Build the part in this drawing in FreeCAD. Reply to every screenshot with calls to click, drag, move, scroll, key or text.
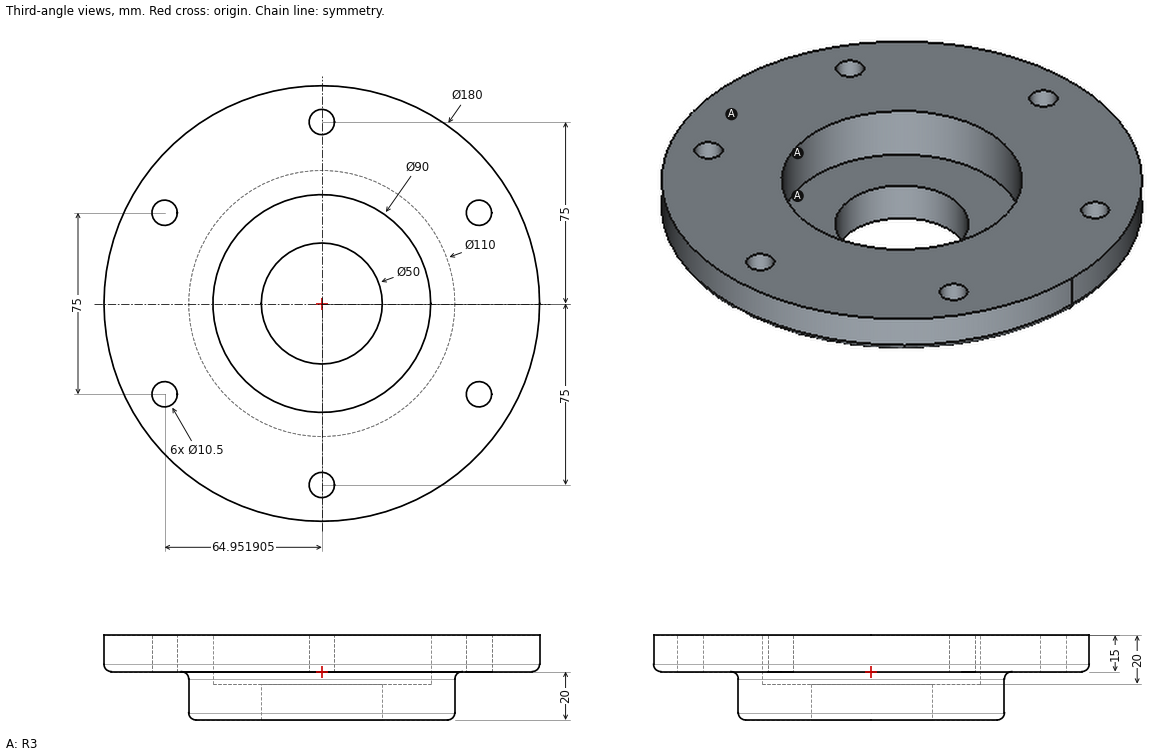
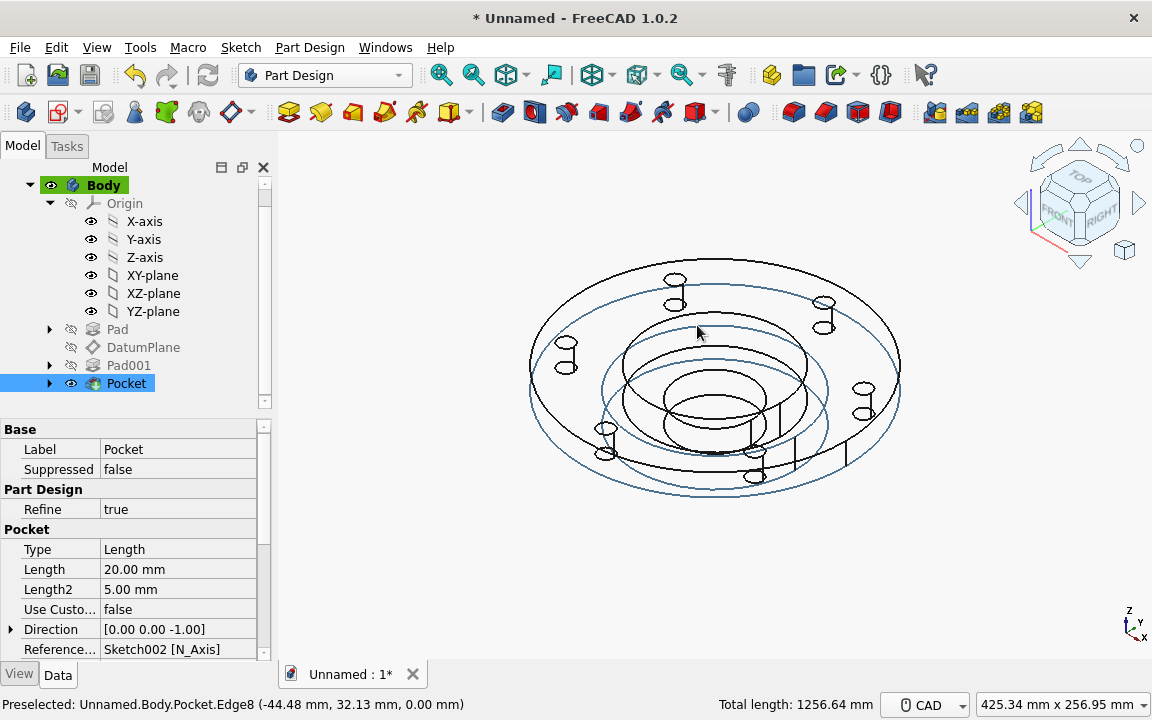
key(v)
key(1)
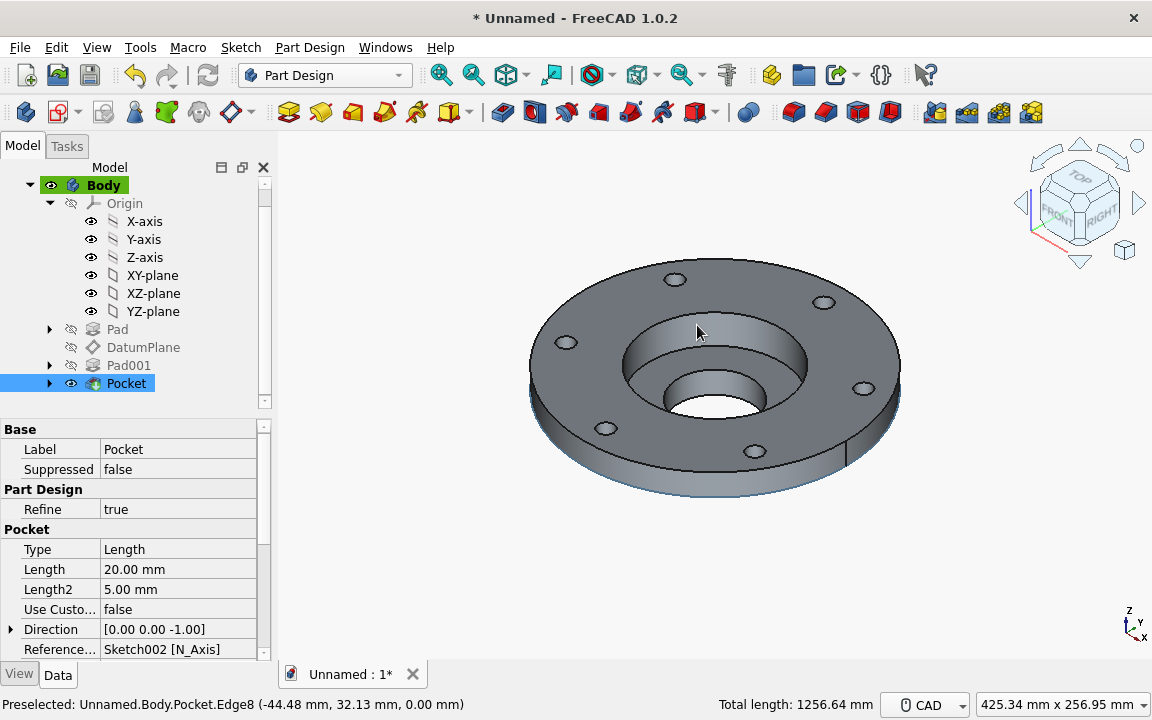
click(794, 112)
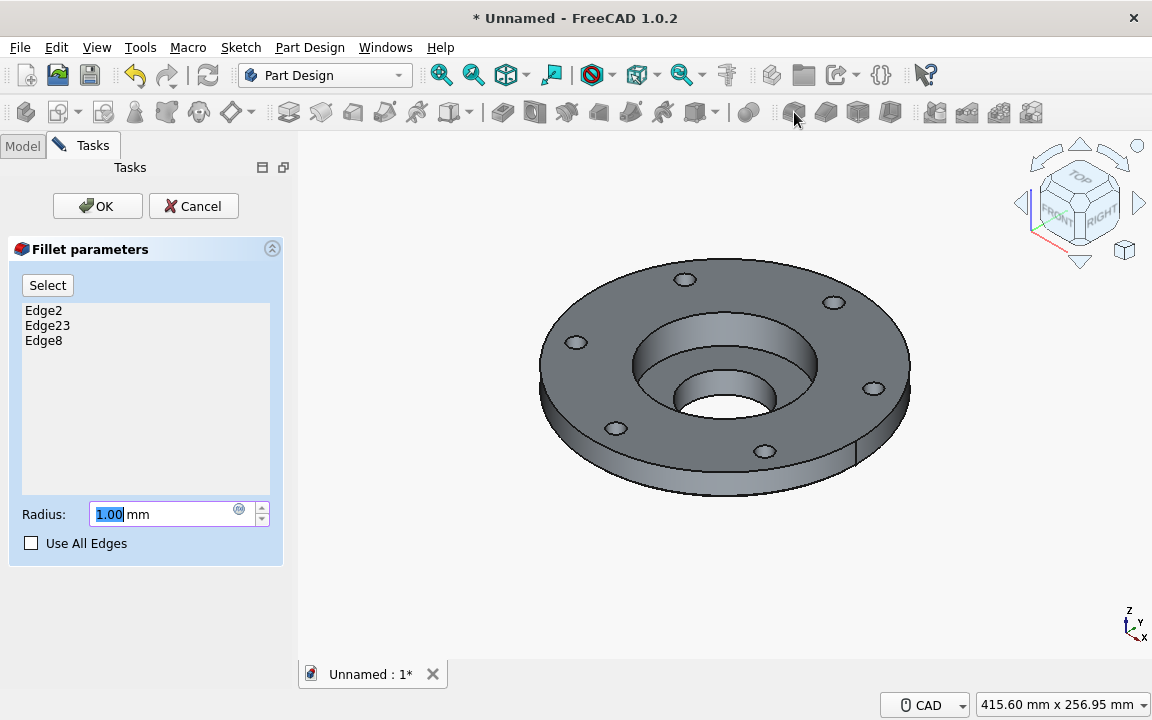
text(3)
key(Tab)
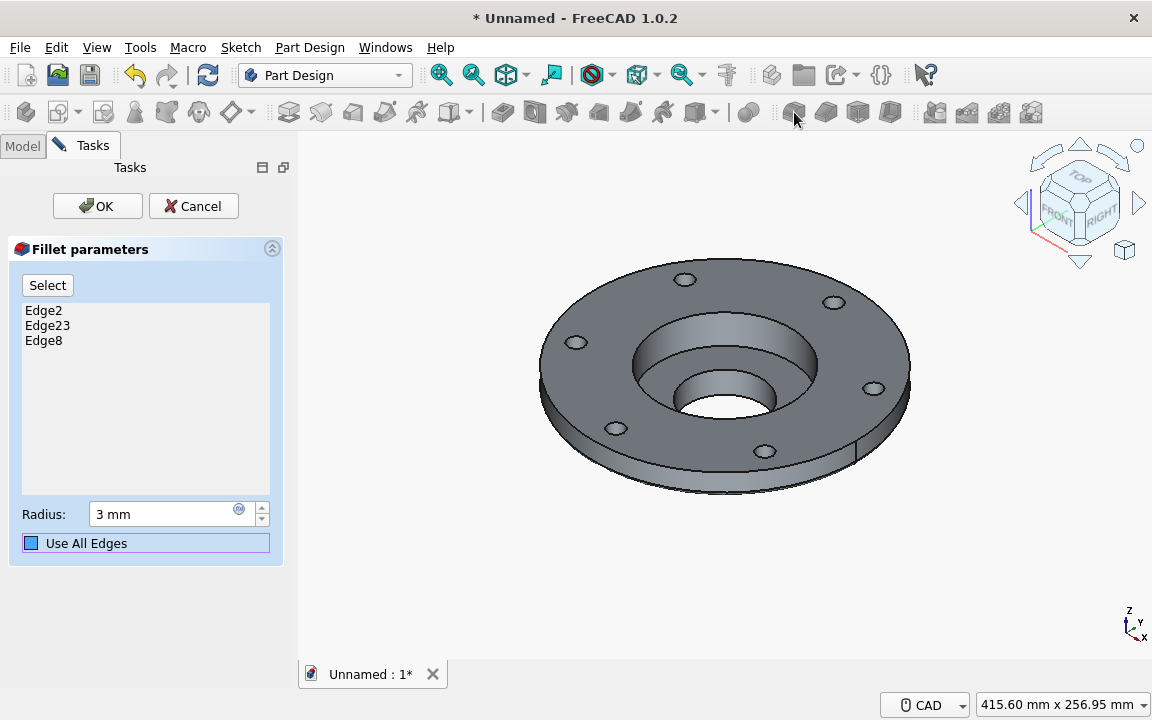
click(98, 206)